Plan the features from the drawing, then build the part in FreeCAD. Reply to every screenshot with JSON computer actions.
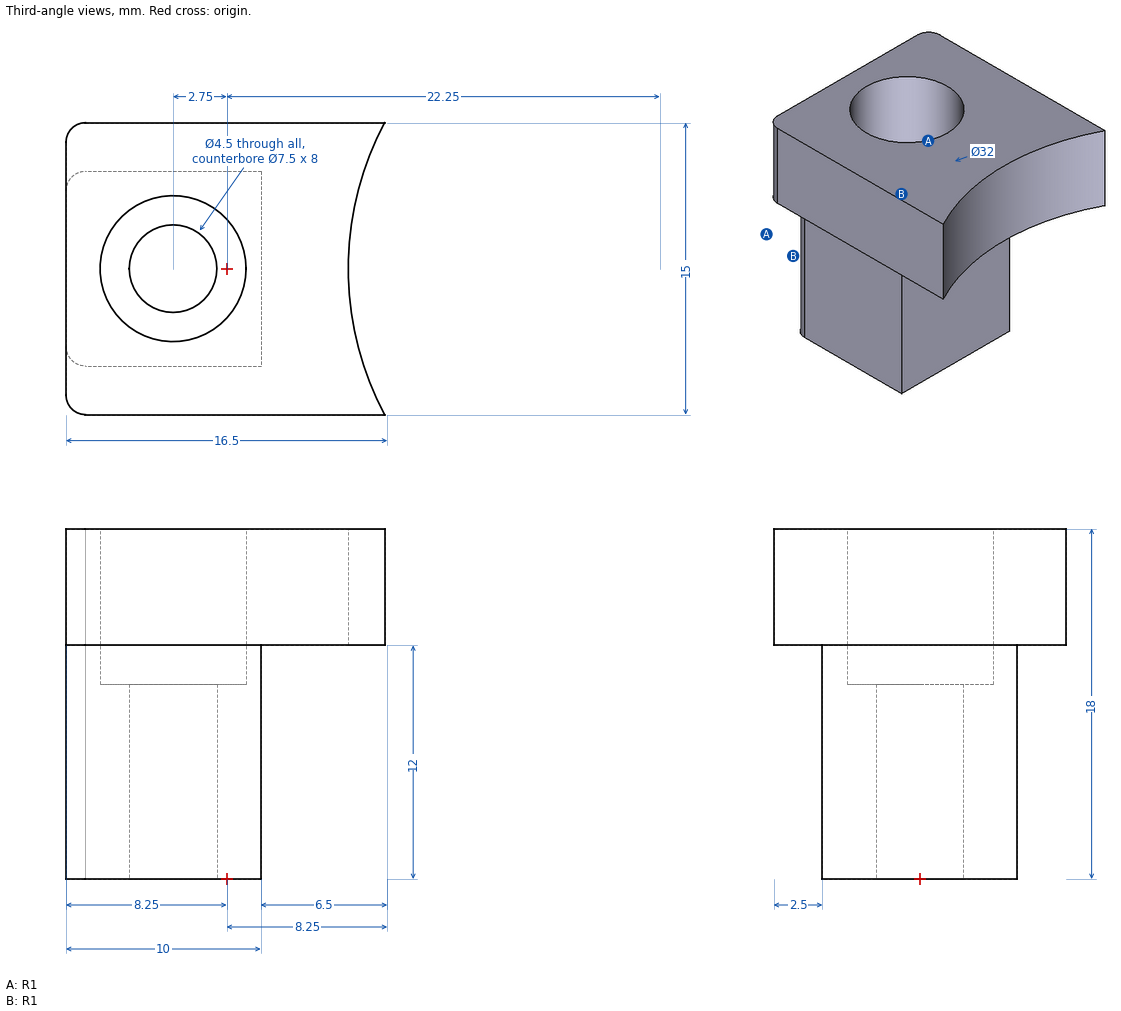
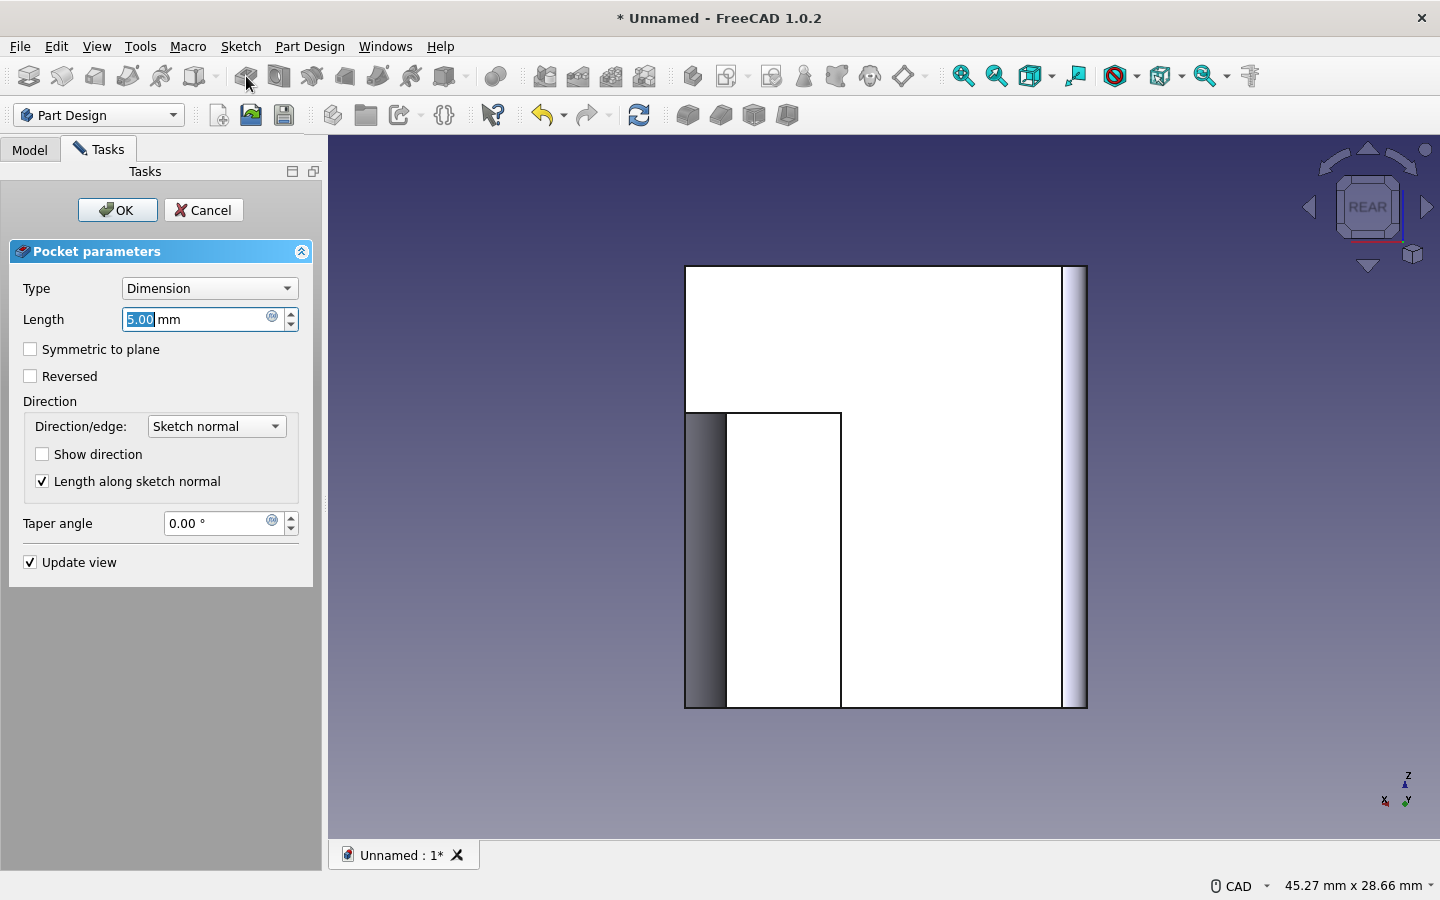
{"action": "left_click", "coordinate": [210, 288]}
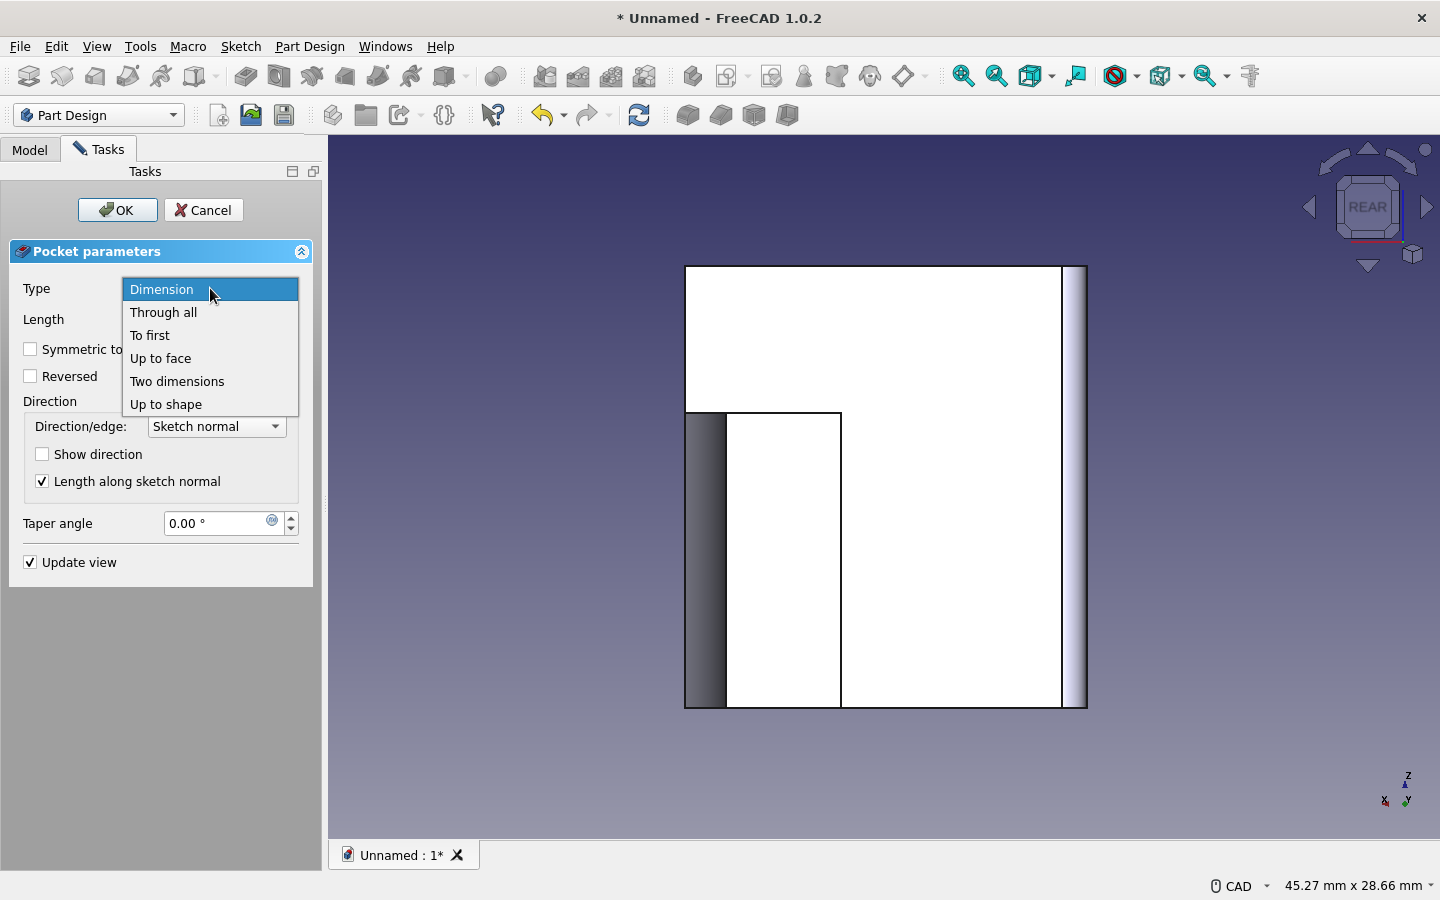
{"action": "left_click", "coordinate": [208, 312]}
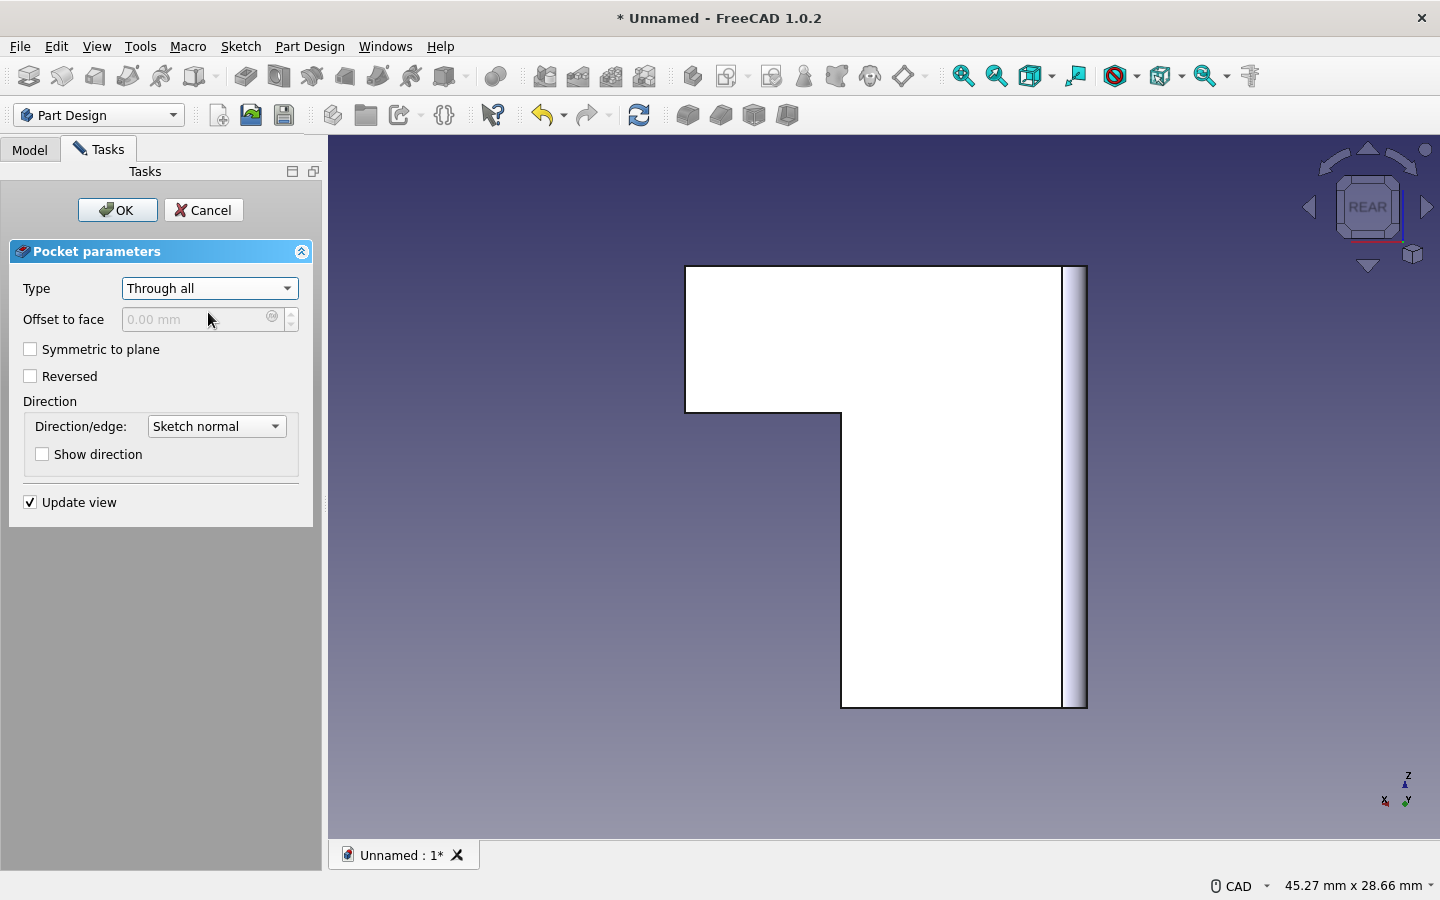
{"action": "left_click", "coordinate": [118, 210]}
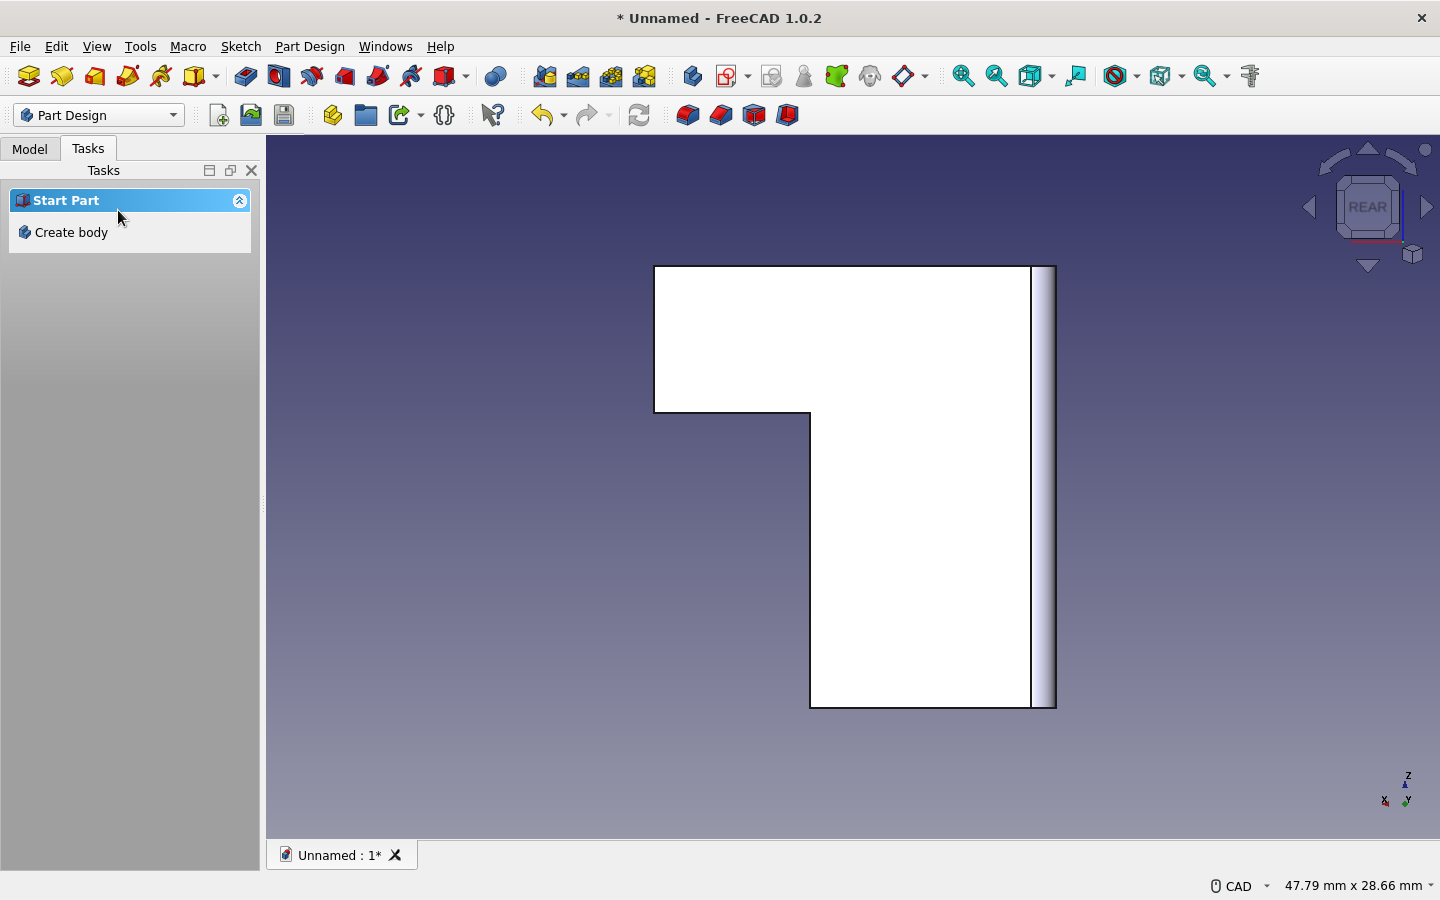
{"action": "key", "text": "0"}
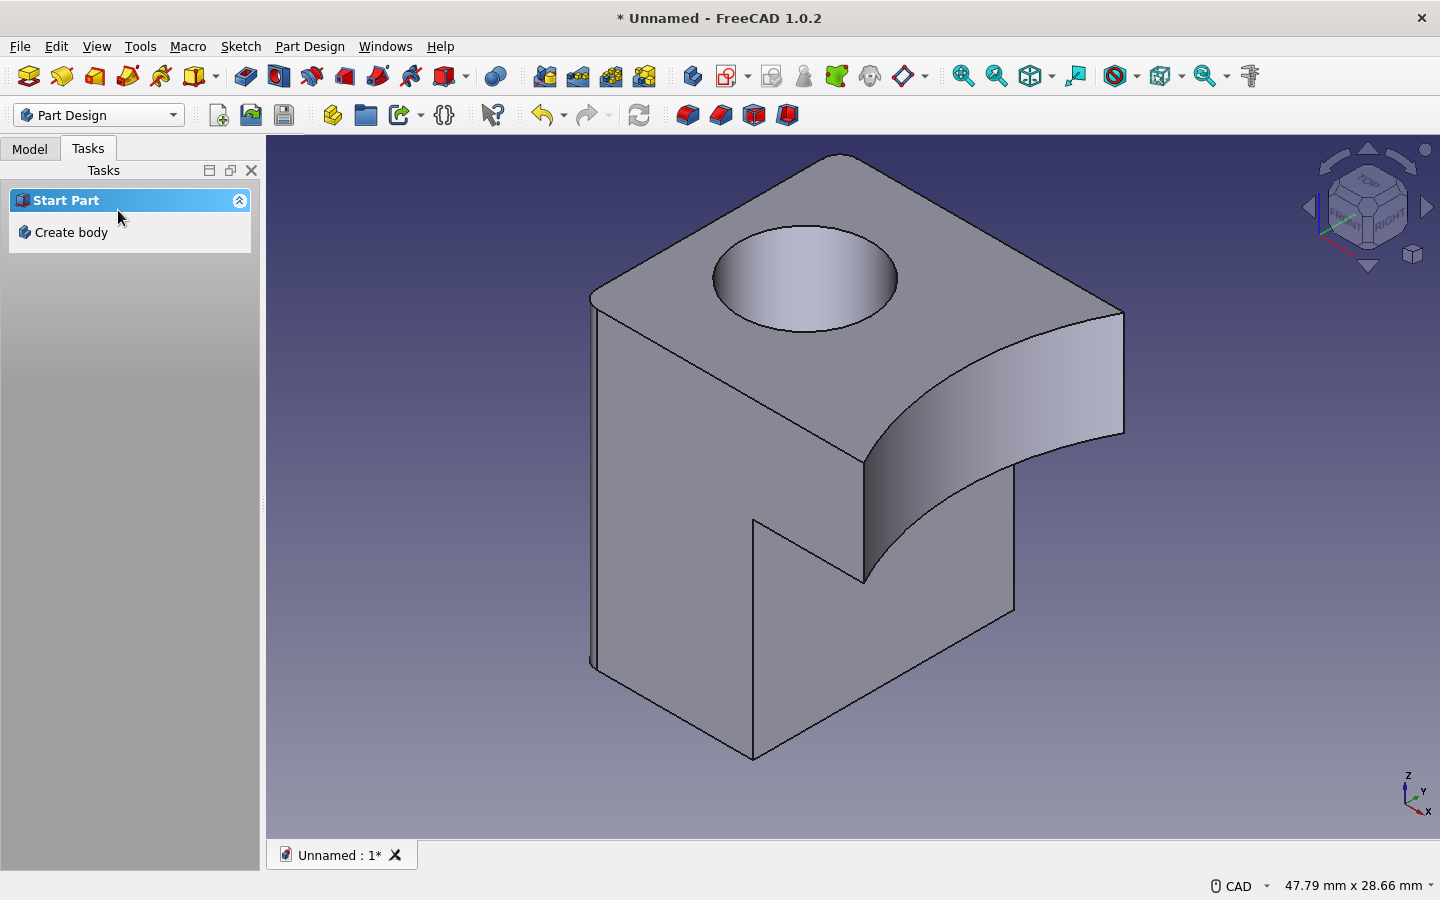
{"action": "left_click", "coordinate": [692, 440]}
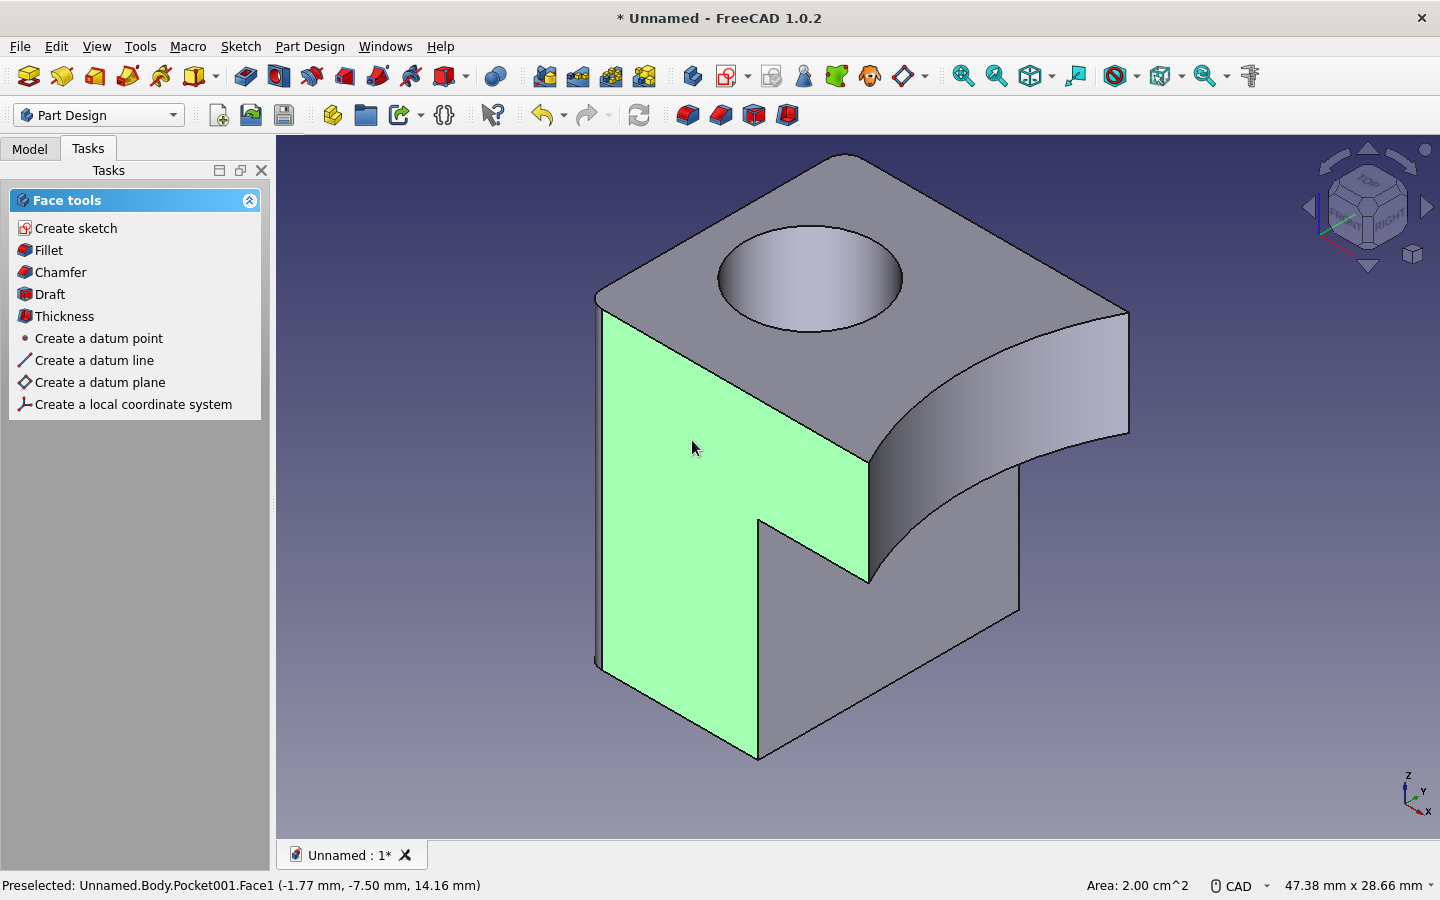
{"action": "left_click", "coordinate": [726, 76]}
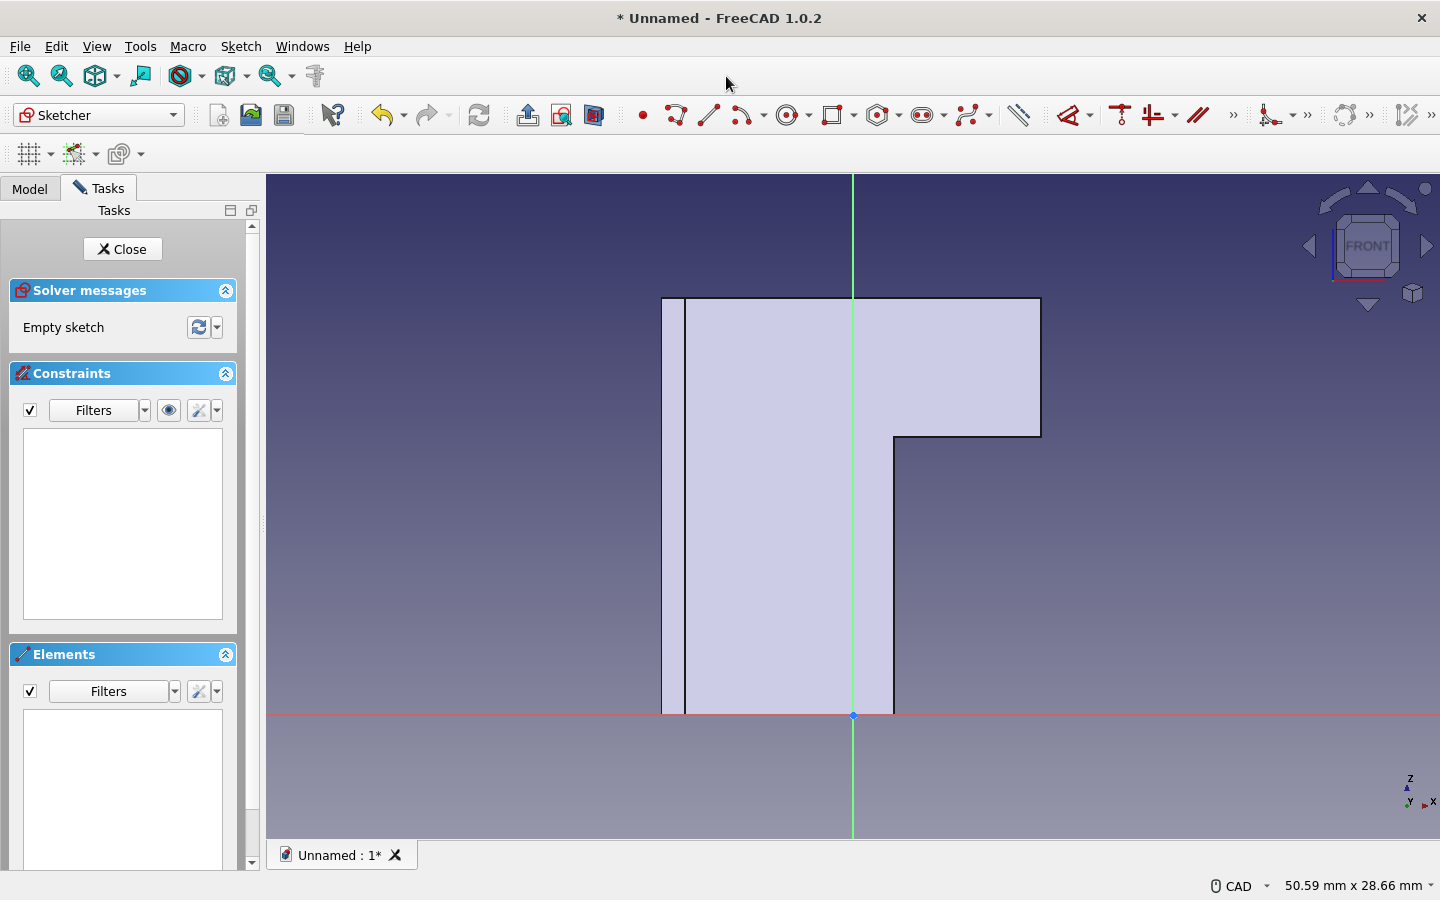
{"action": "scroll", "coordinate": [764, 718], "scroll_direction": "up", "scroll_amount": 2}